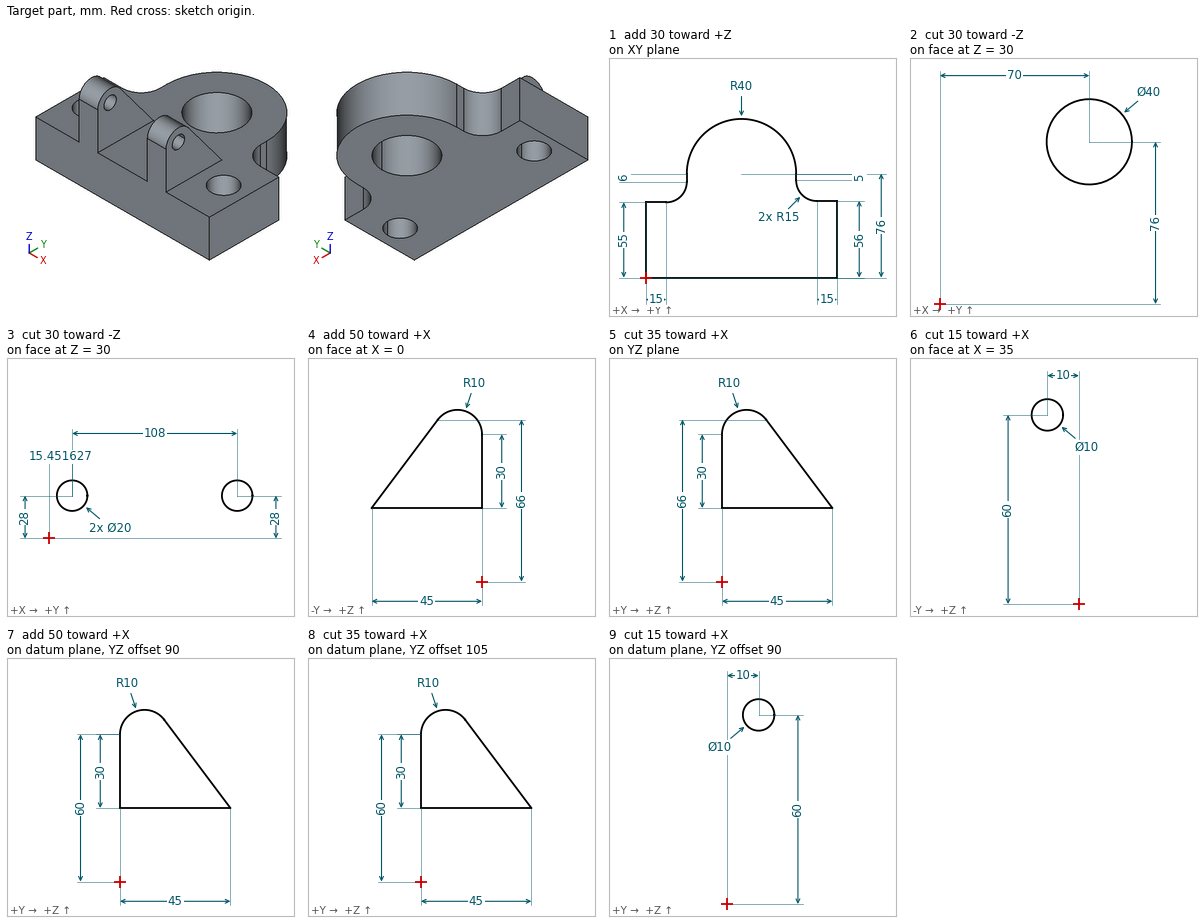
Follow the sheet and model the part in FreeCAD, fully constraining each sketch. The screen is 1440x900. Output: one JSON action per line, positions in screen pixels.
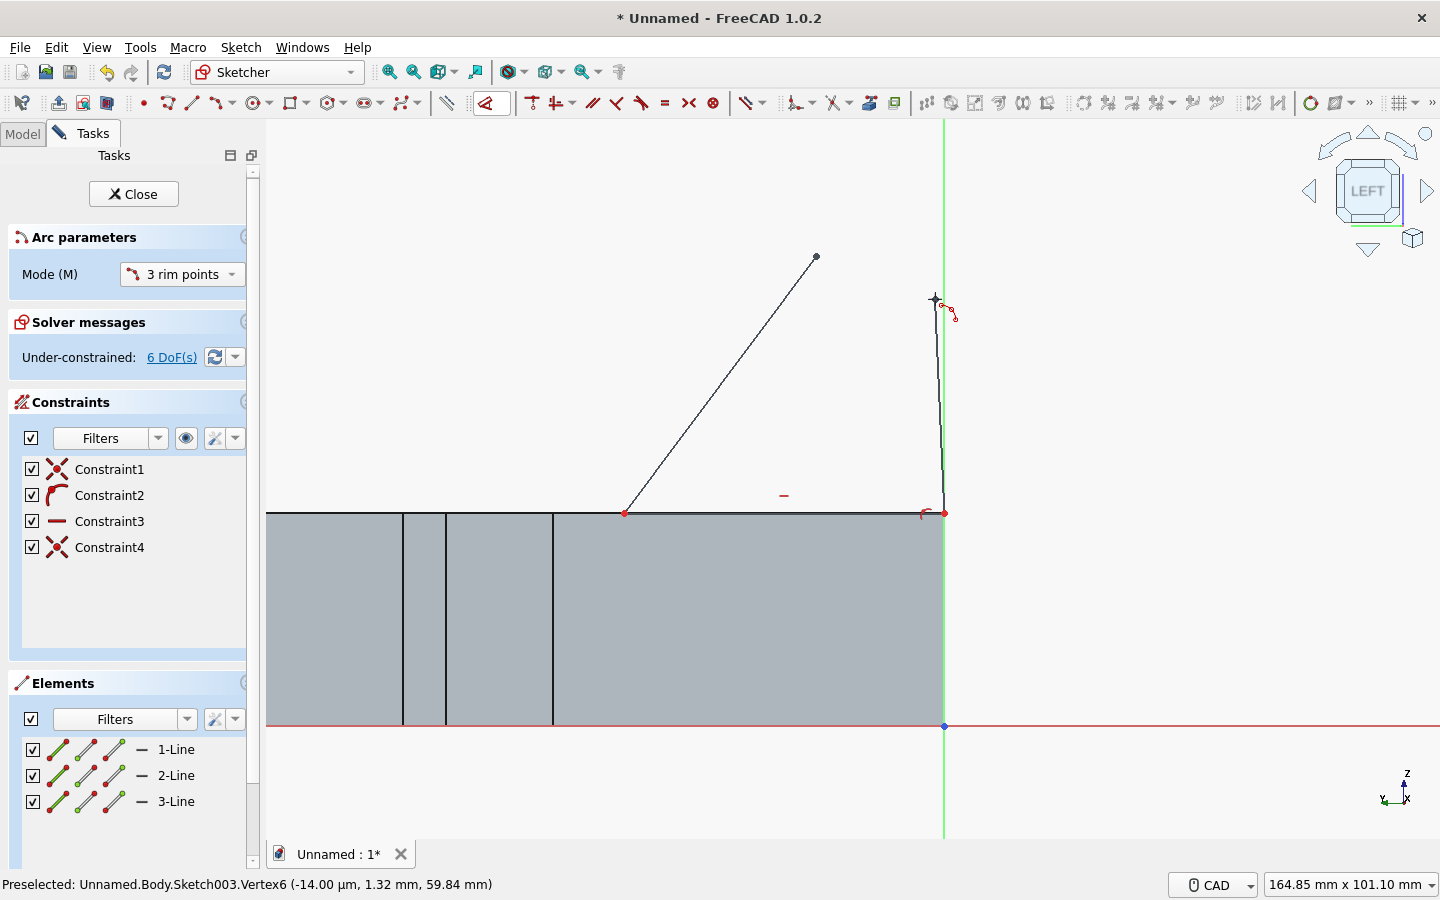
{"action": "left_click", "coordinate": [935, 300]}
{"action": "left_click", "coordinate": [816, 257]}
{"action": "left_click", "coordinate": [896, 231]}
{"action": "key", "text": "Escape"}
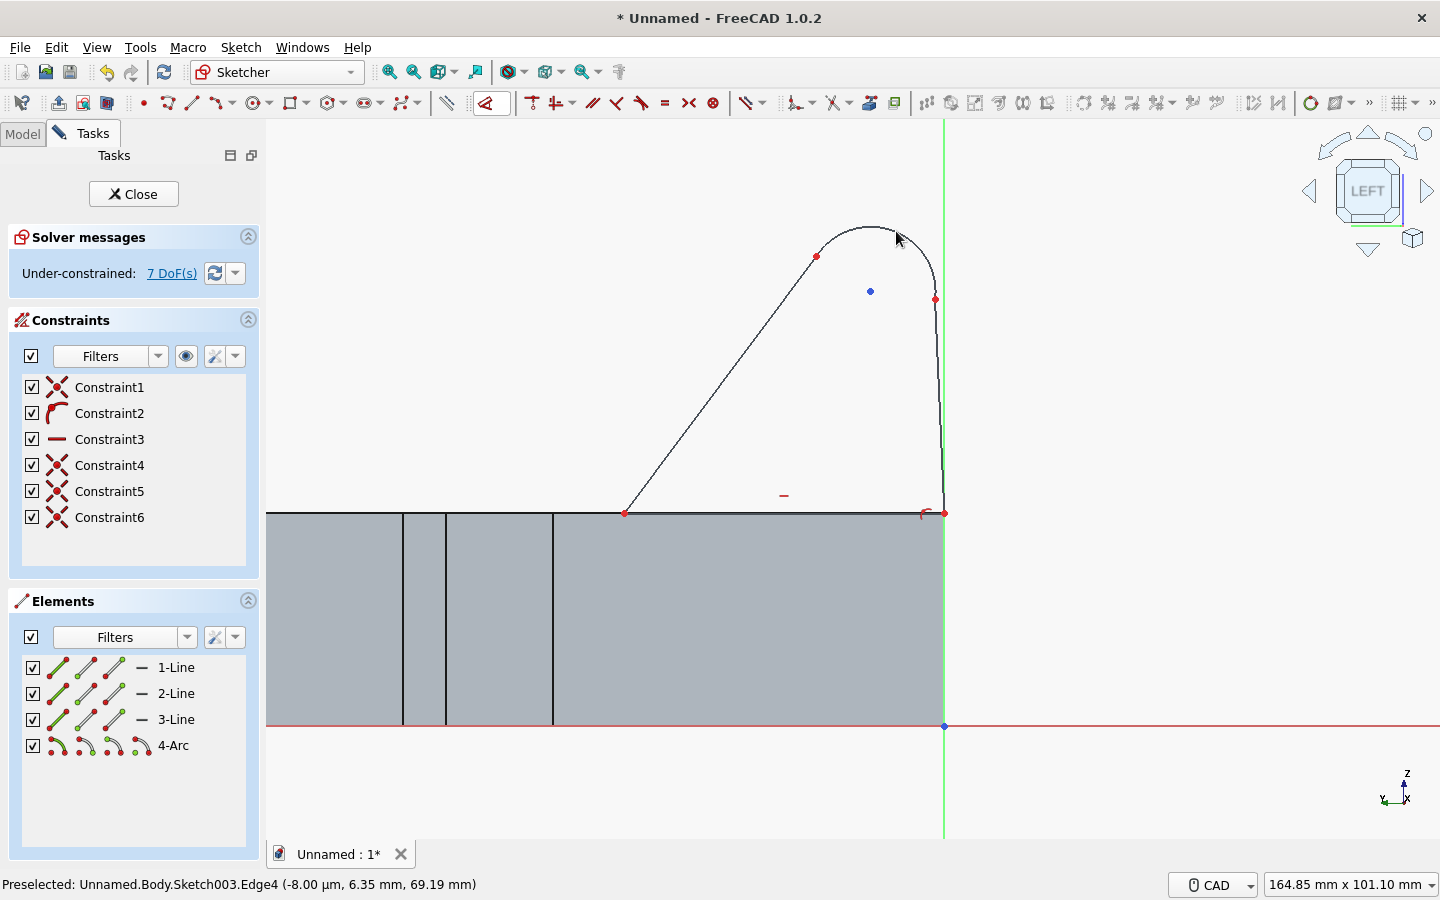
{"action": "left_click", "coordinate": [758, 334]}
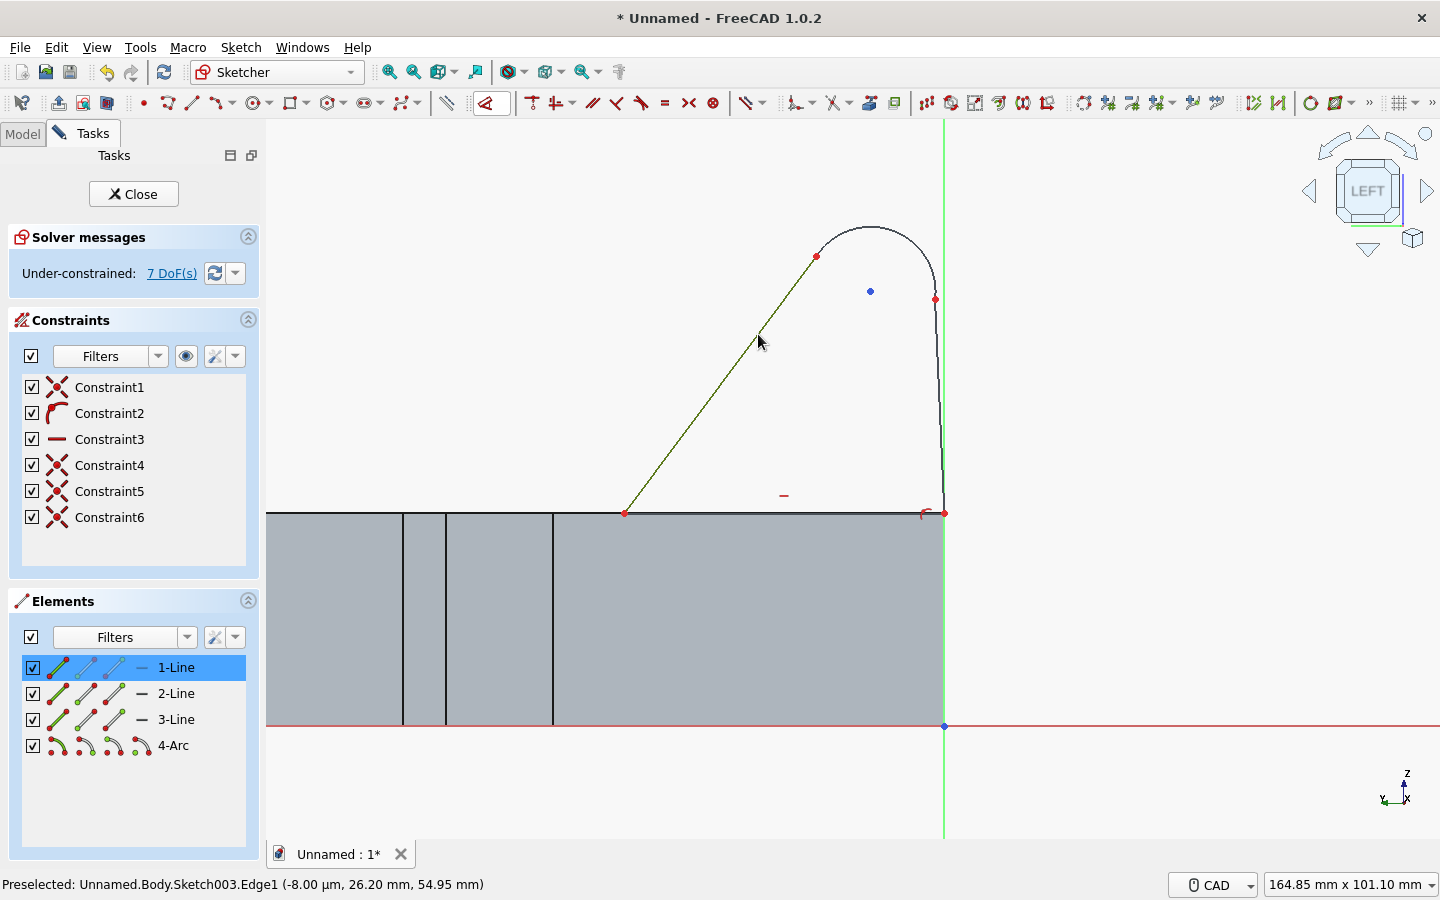
{"action": "left_click", "coordinate": [921, 251]}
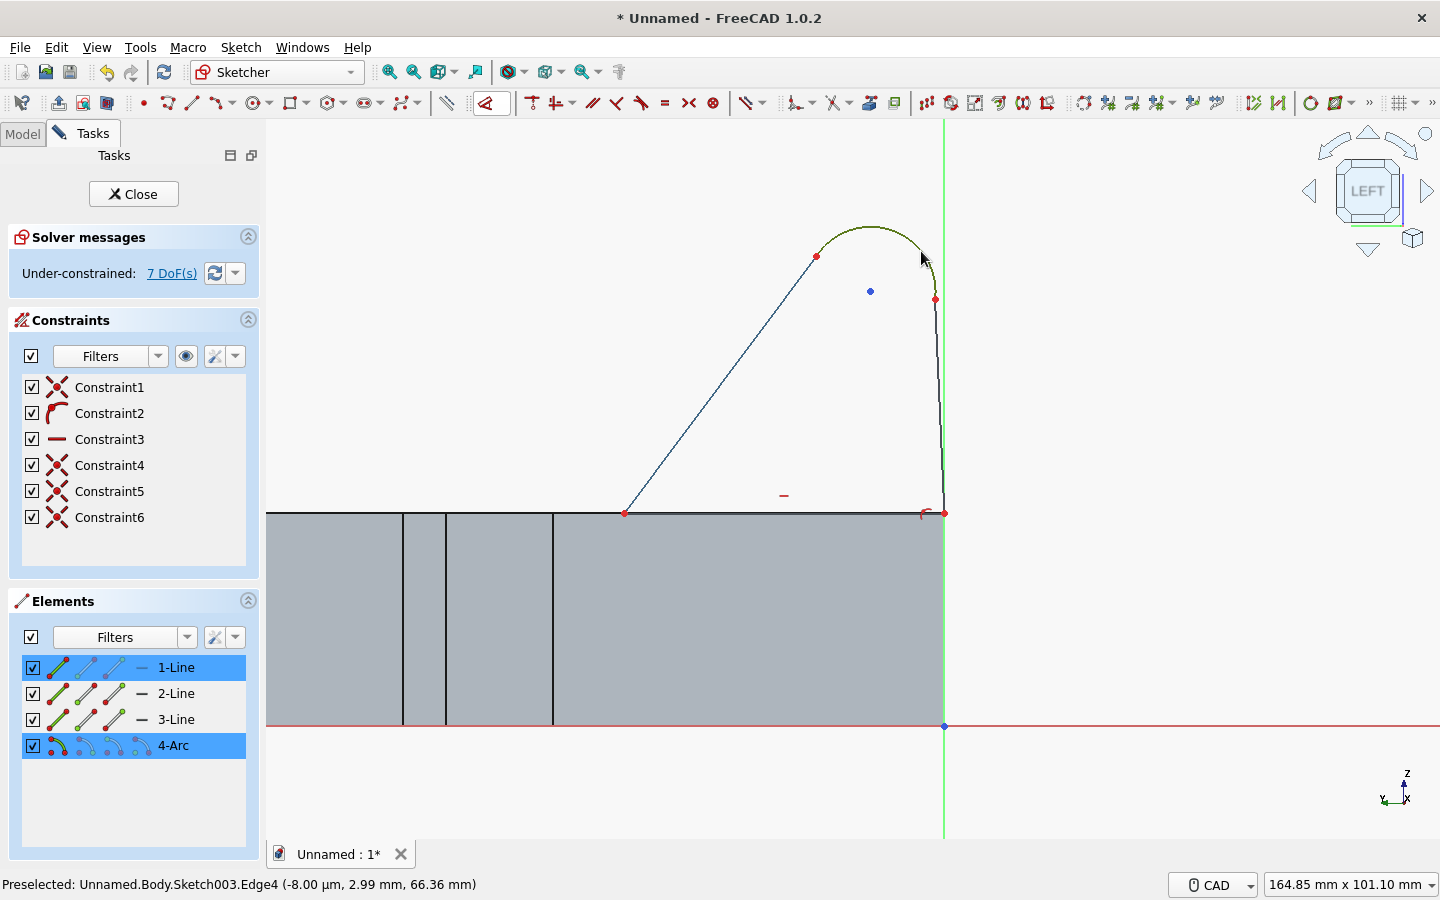
{"action": "left_click", "coordinate": [642, 104]}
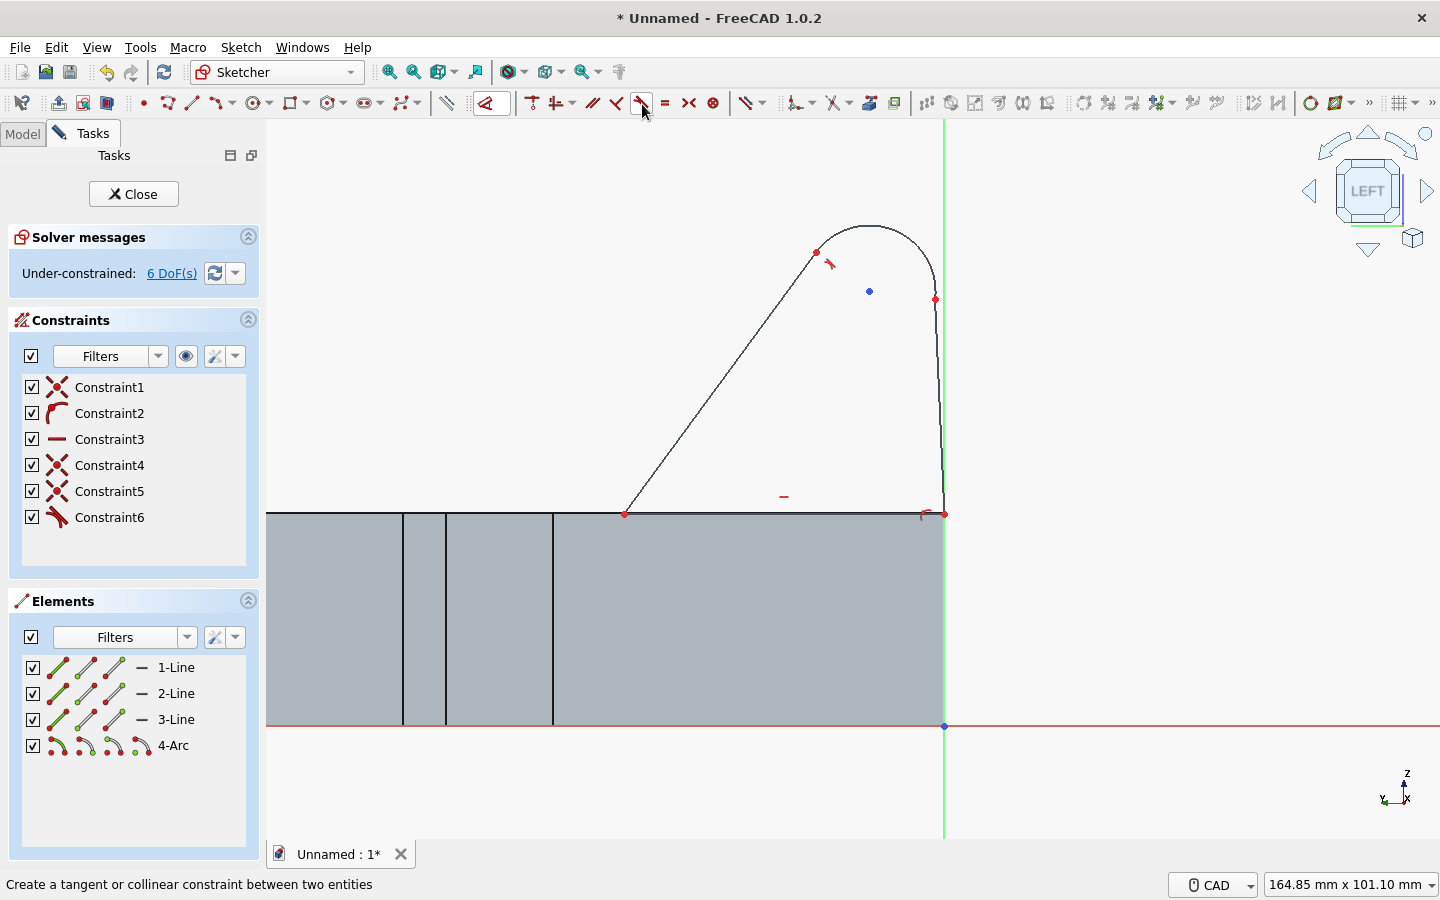
{"action": "left_click", "coordinate": [942, 450]}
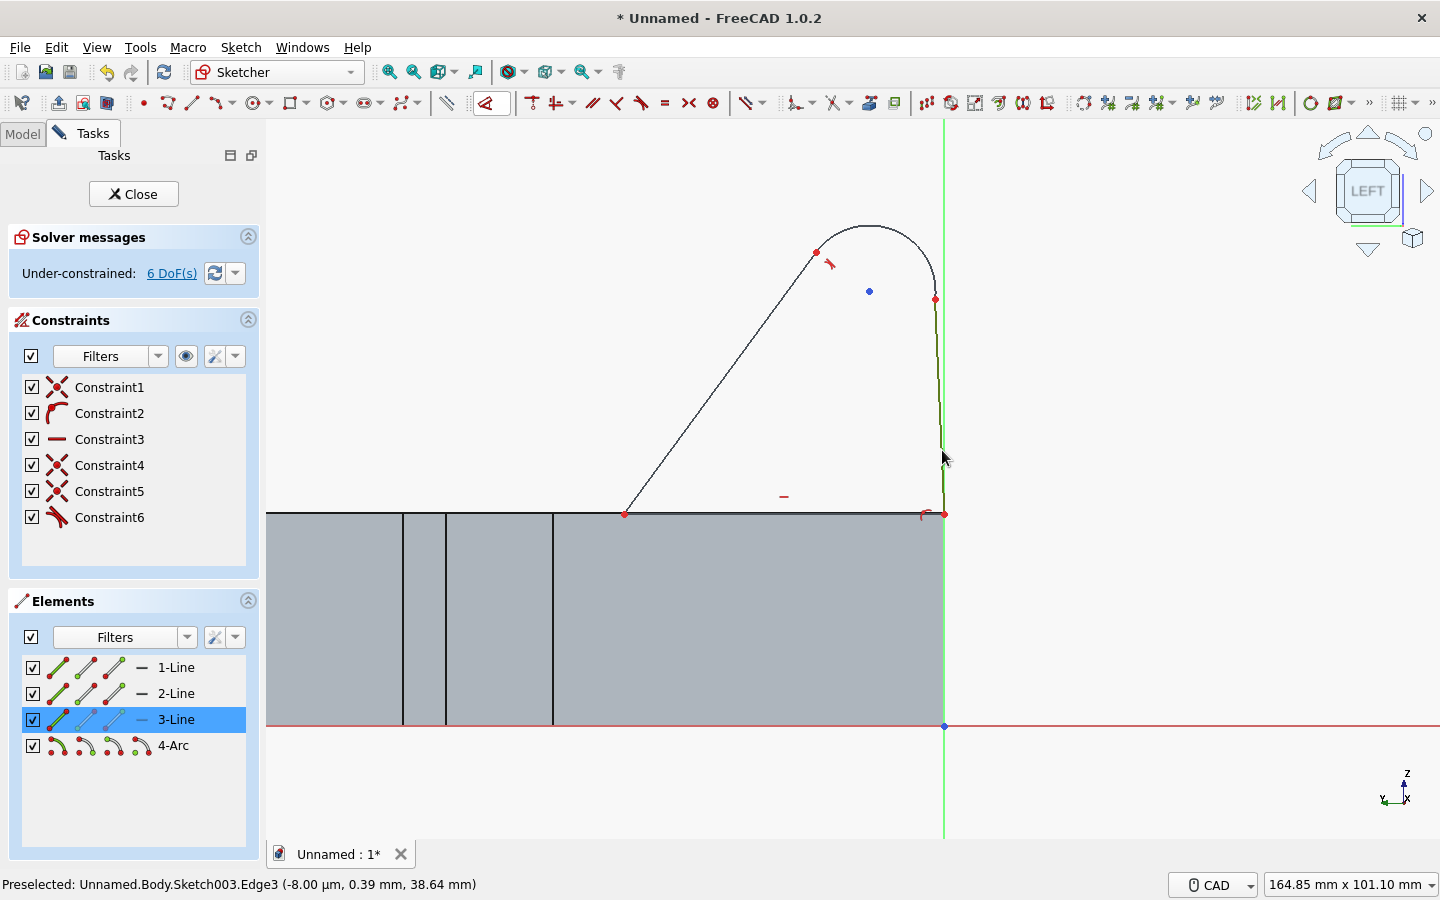
{"action": "left_click", "coordinate": [921, 251]}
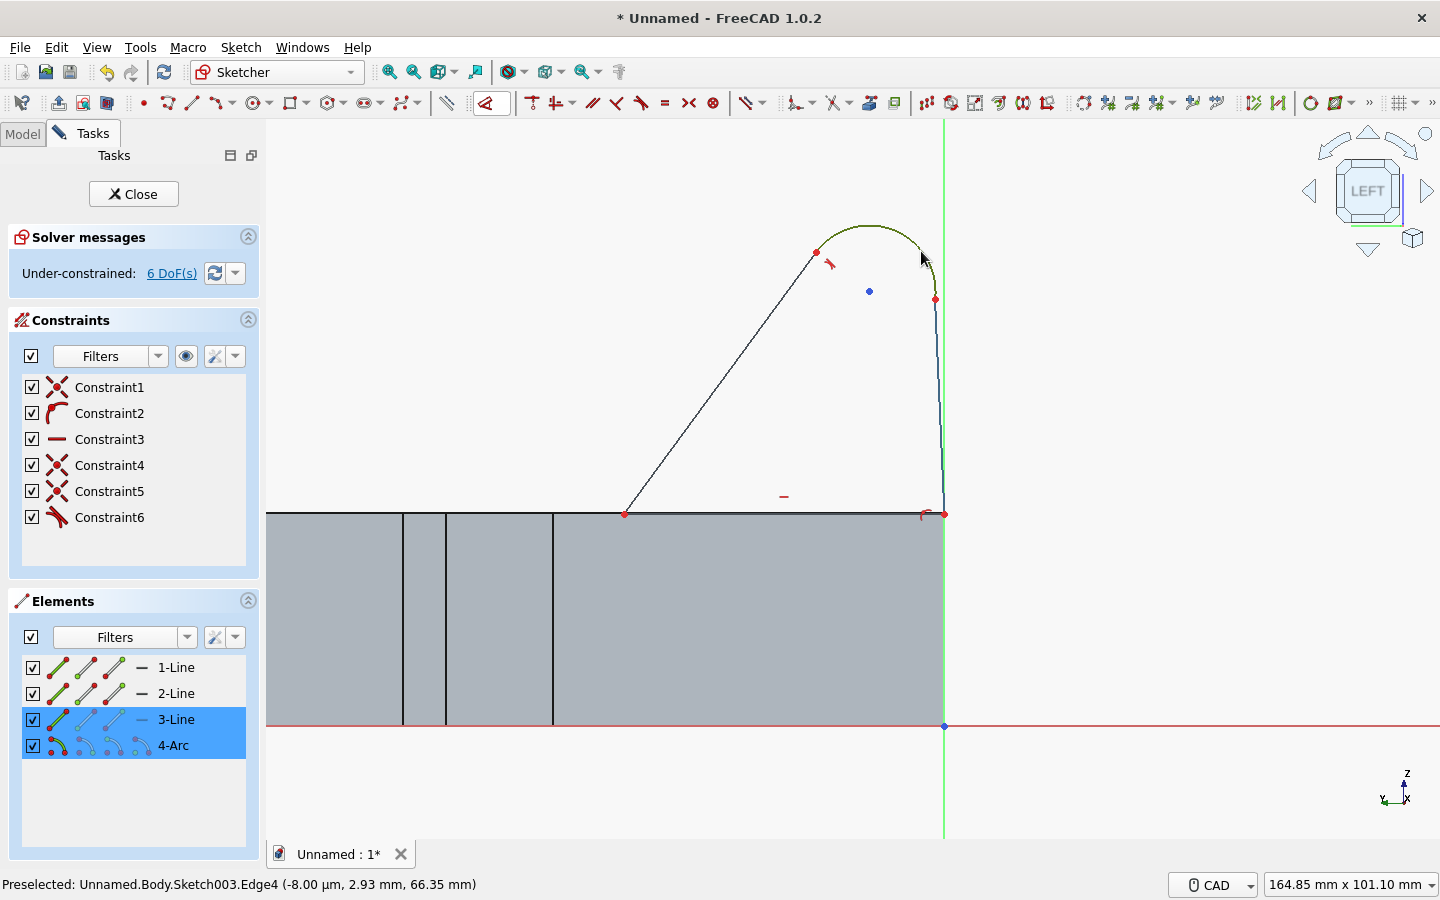
{"action": "key", "text": "t"}